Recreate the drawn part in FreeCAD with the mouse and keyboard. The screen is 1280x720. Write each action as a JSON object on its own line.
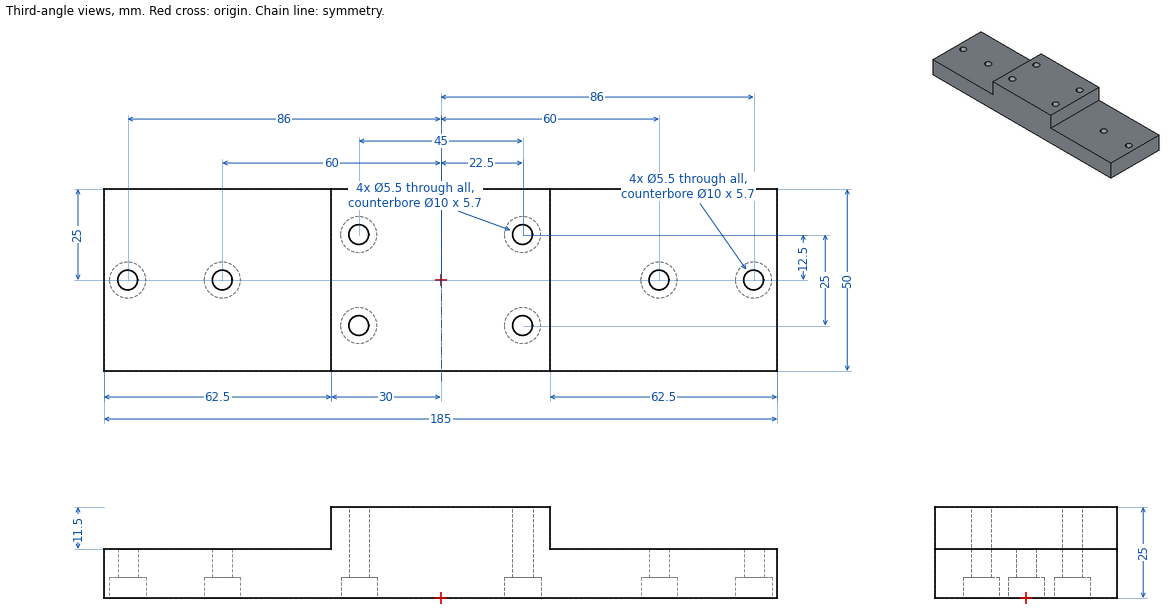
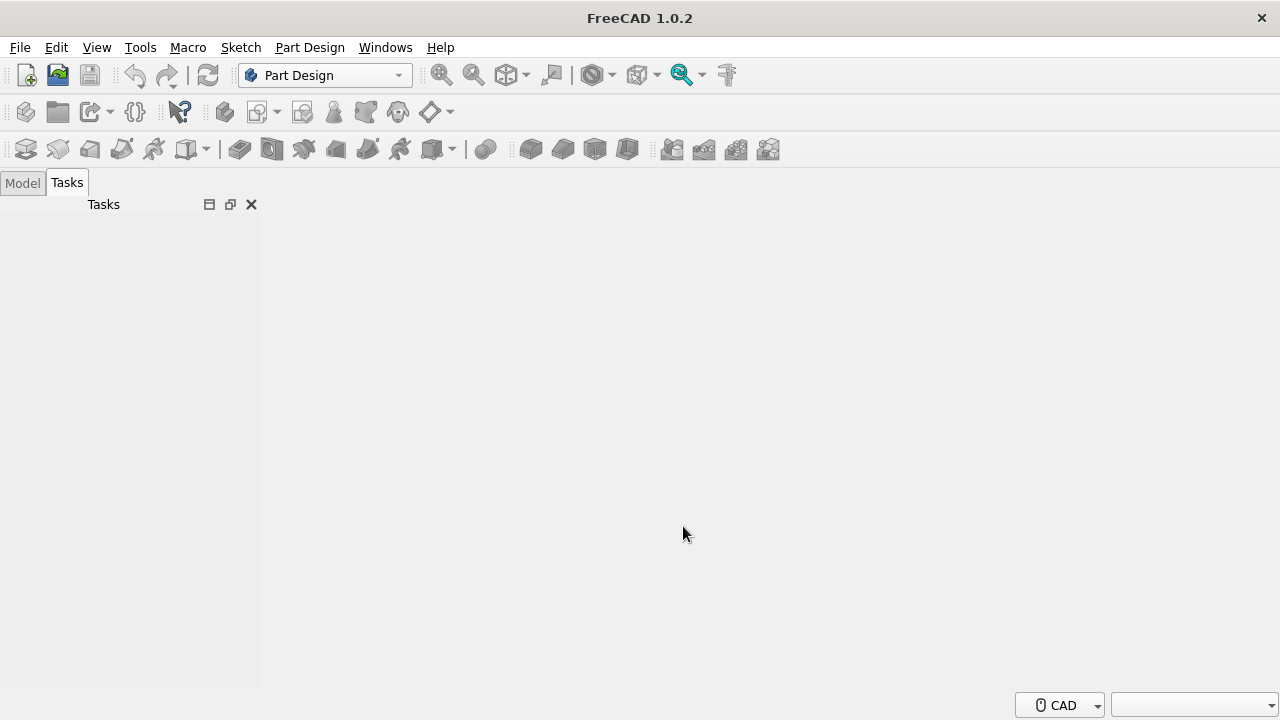
{"action": "key", "text": "ctrl+n"}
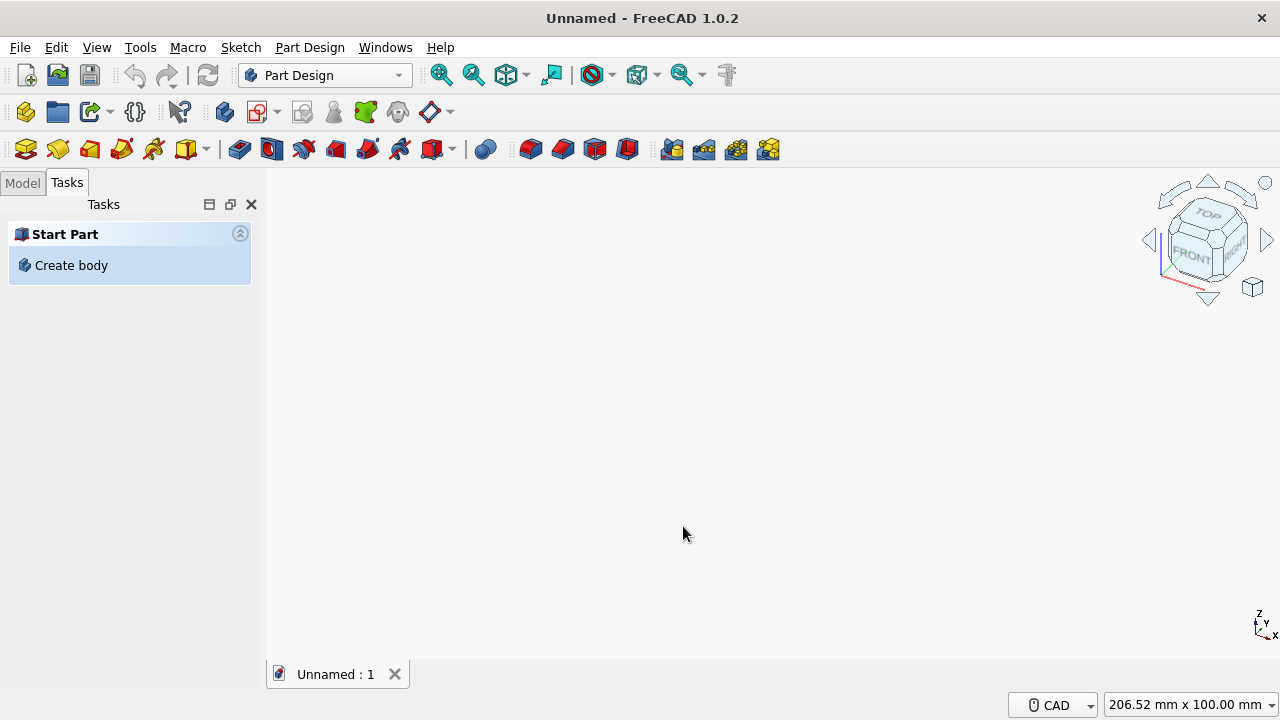
{"action": "left_click", "coordinate": [258, 112]}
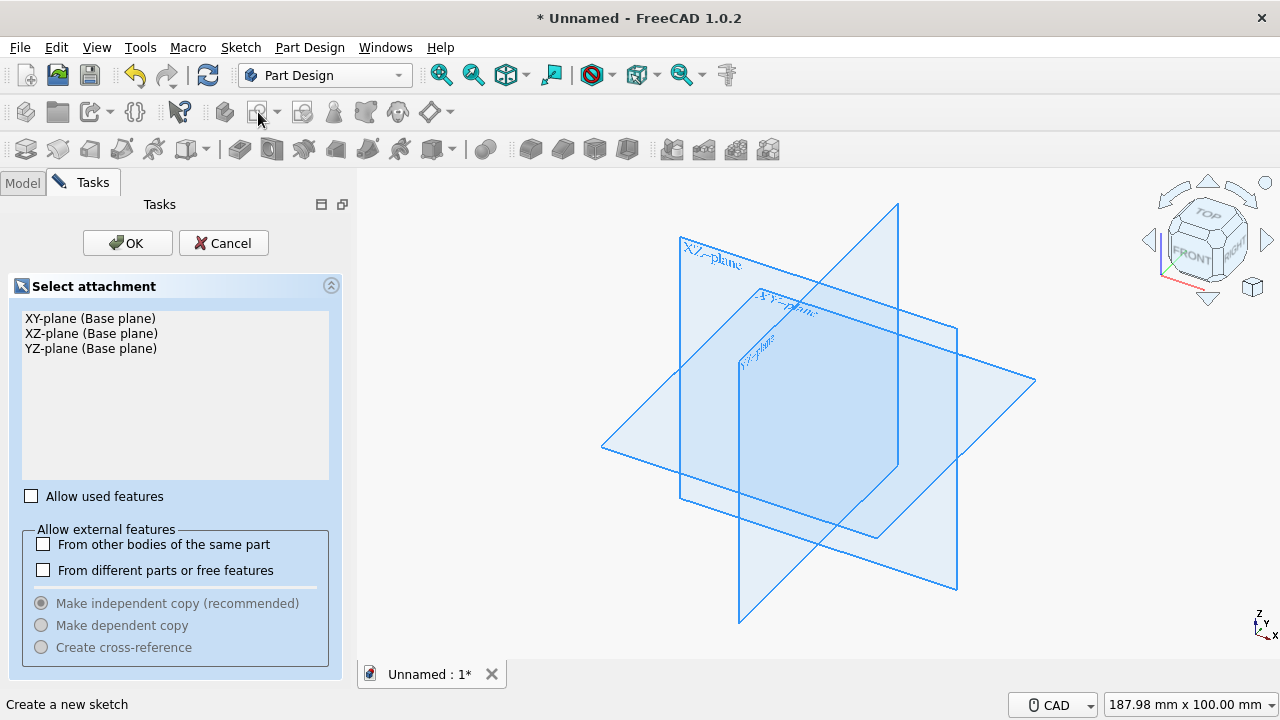
{"action": "left_click", "coordinate": [82, 318]}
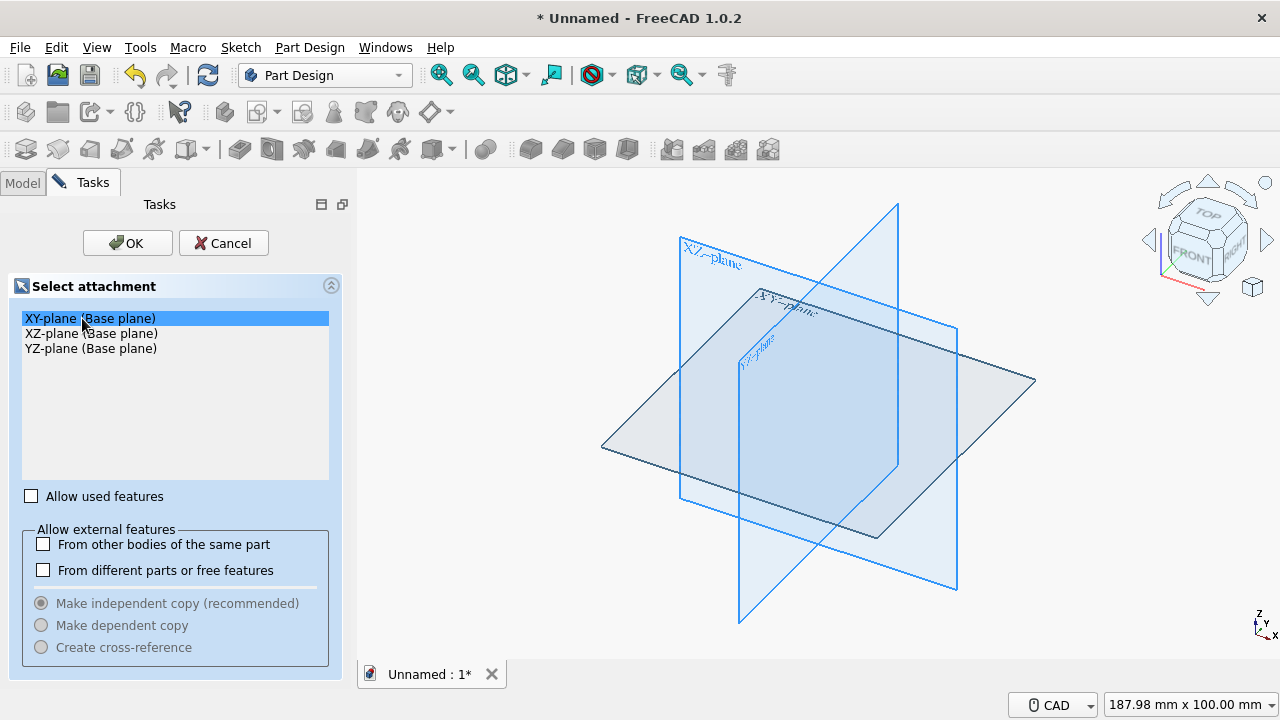
{"action": "left_click", "coordinate": [128, 243]}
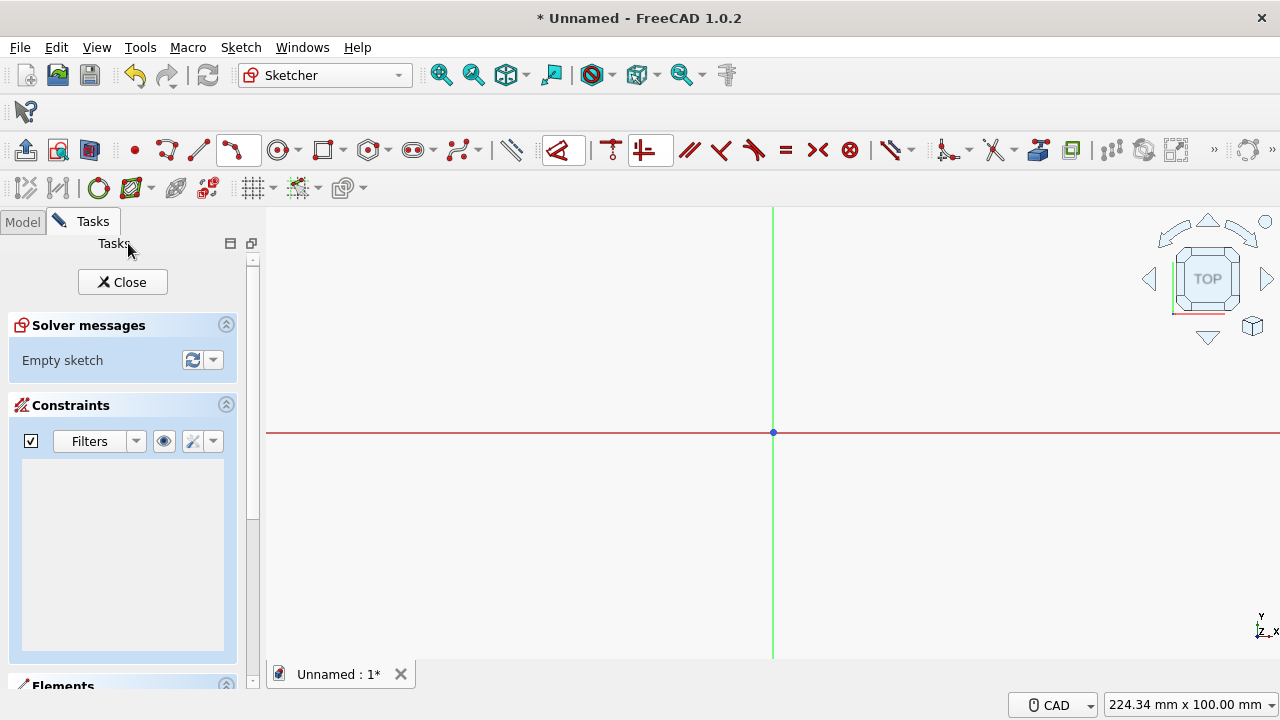
{"action": "scroll", "coordinate": [565, 433], "scroll_direction": "down", "scroll_amount": 2}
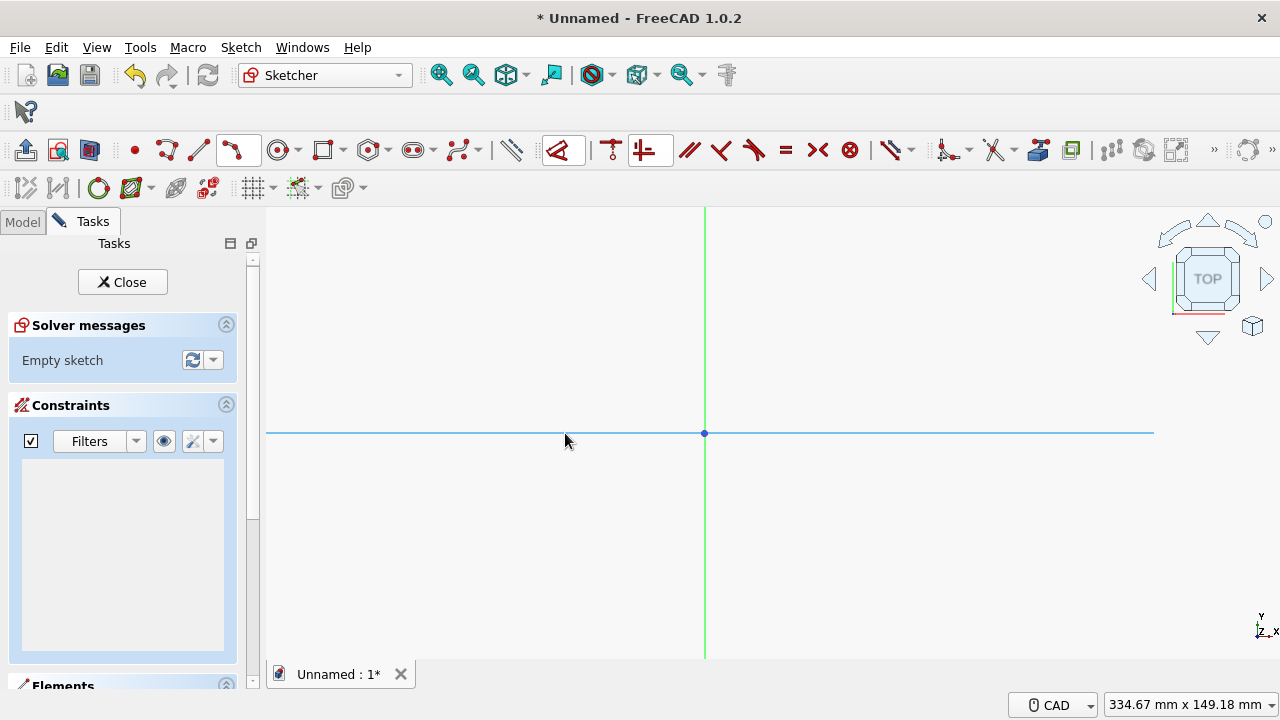
{"action": "key", "text": "g v"}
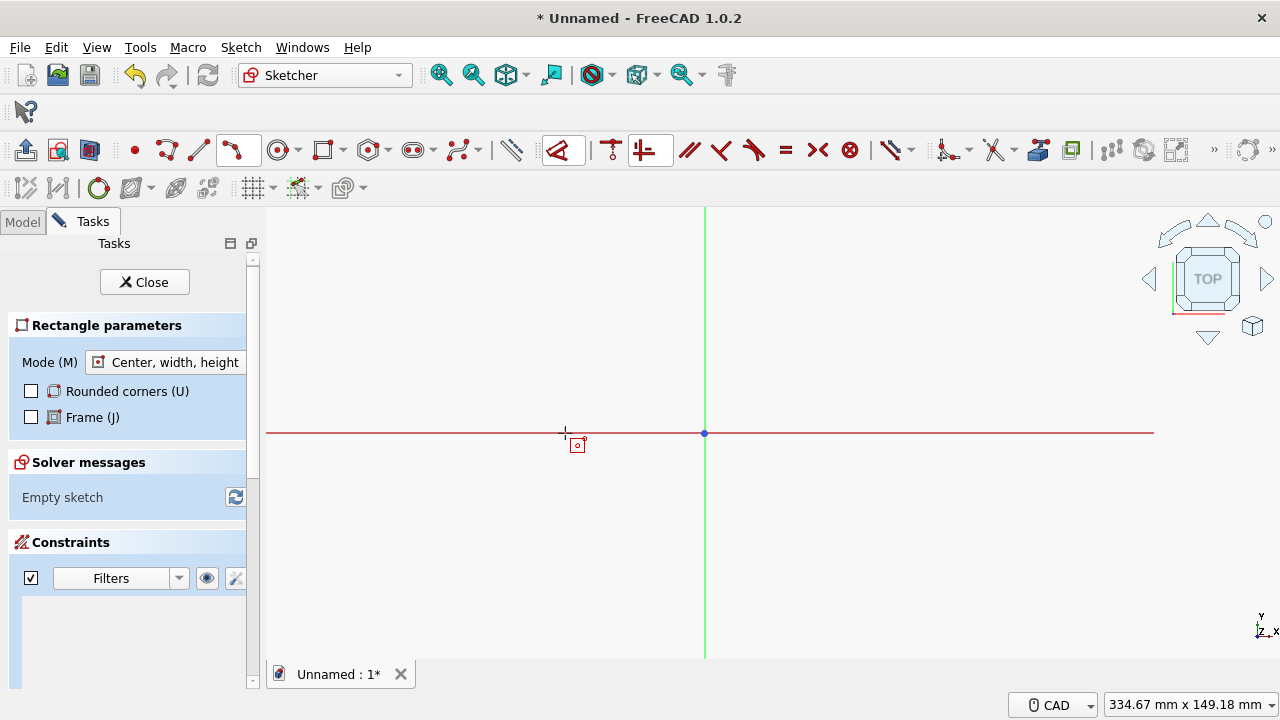
{"action": "left_click", "coordinate": [705, 433]}
{"action": "mouse_move", "coordinate": [985, 357]}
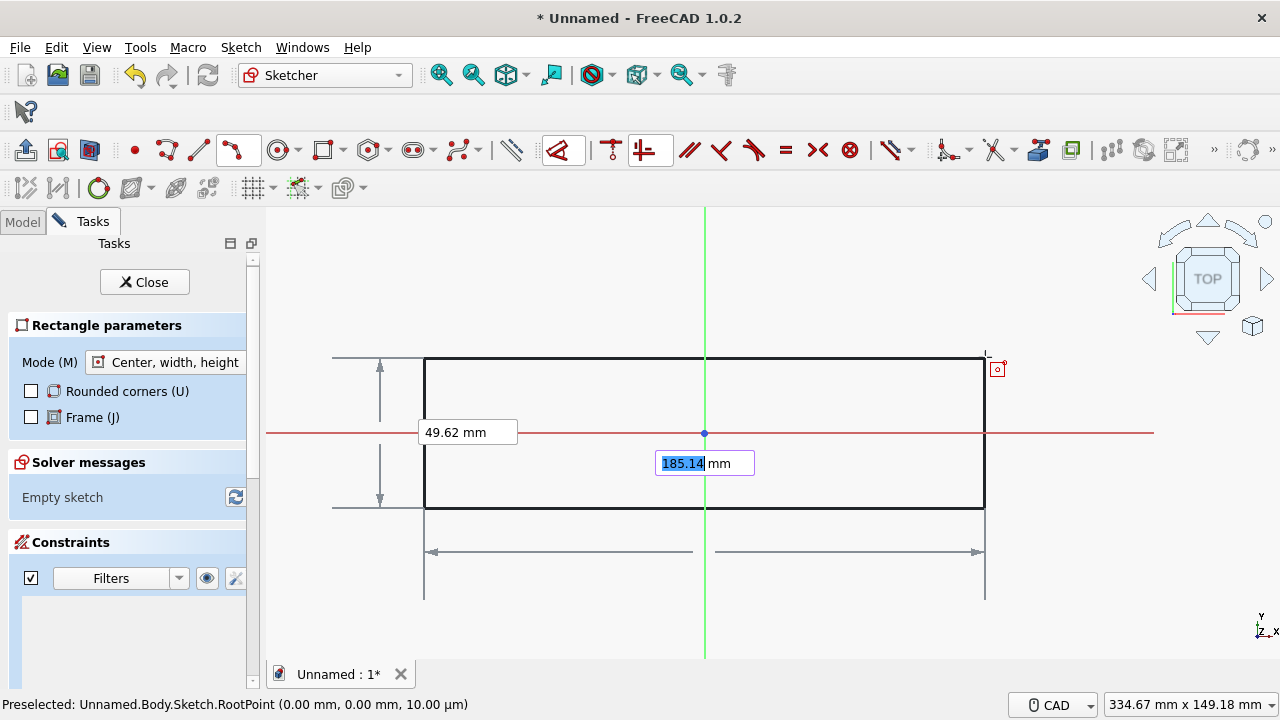
{"action": "type", "text": "185"}
{"action": "key", "text": "Tab"}
{"action": "type", "text": "50"}
{"action": "key", "text": "Return"}
{"action": "key", "text": "Escape"}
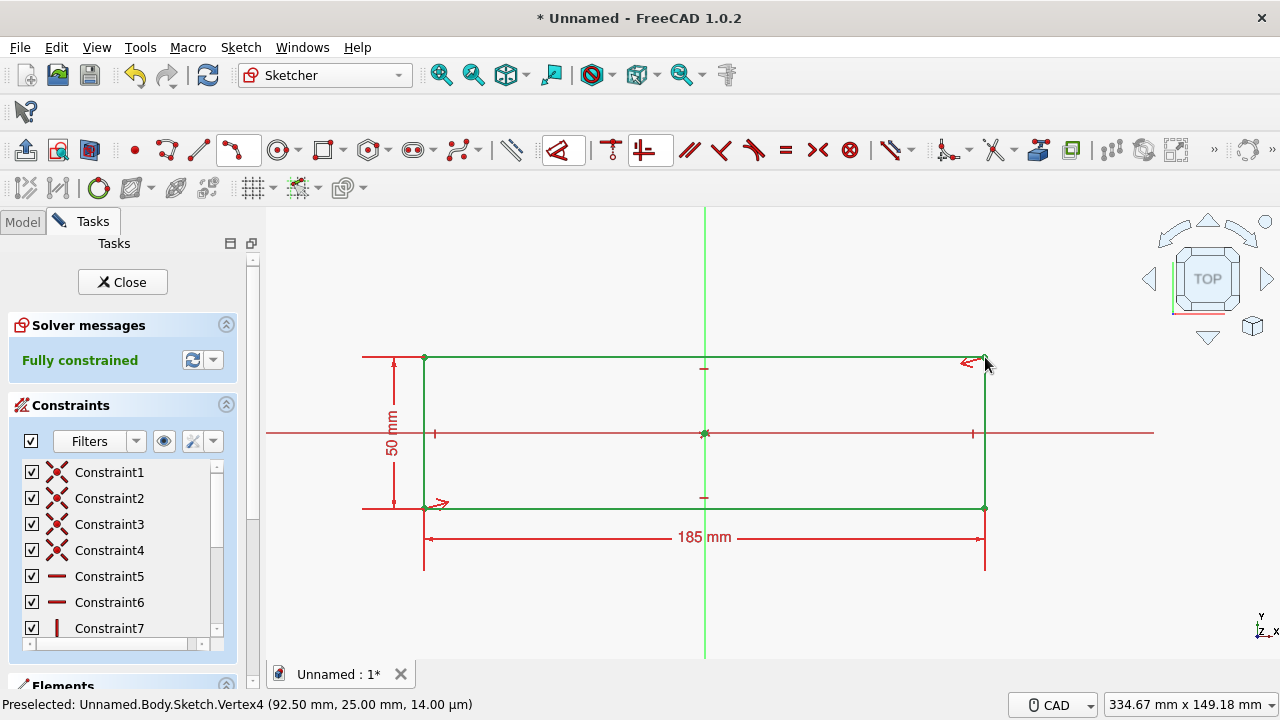
{"action": "left_click", "coordinate": [123, 282]}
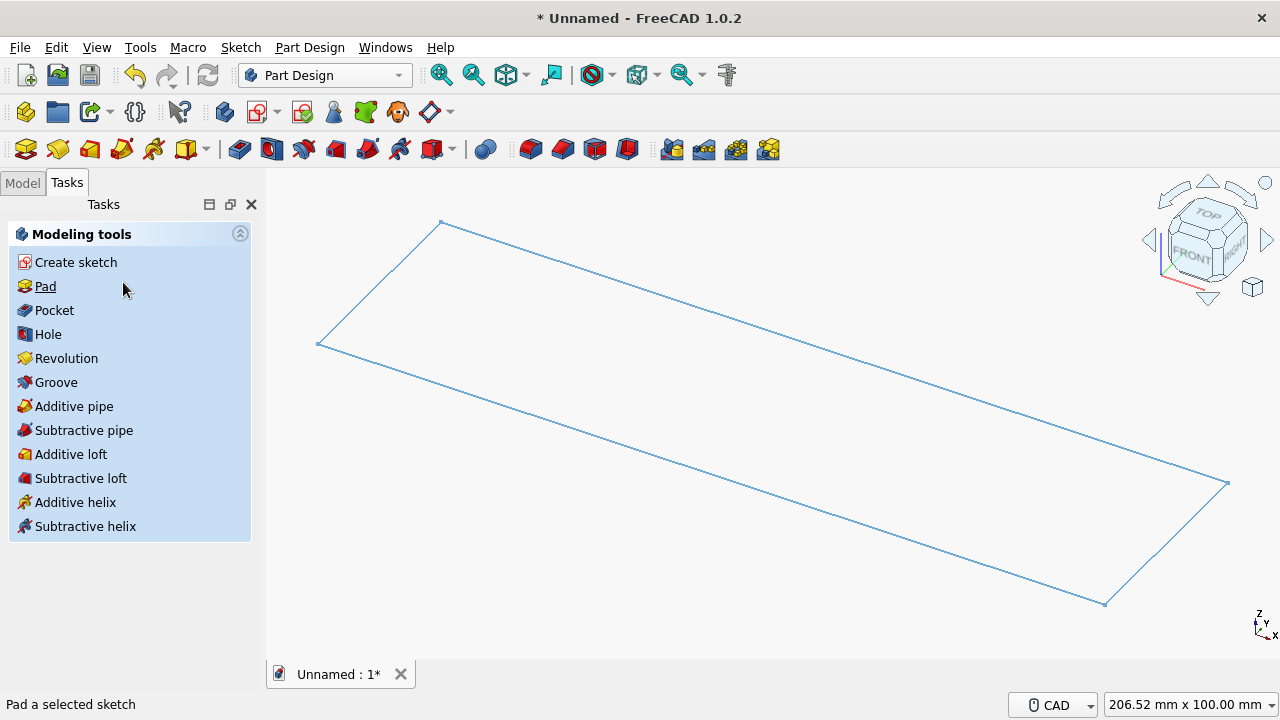
{"action": "left_click", "coordinate": [26, 150]}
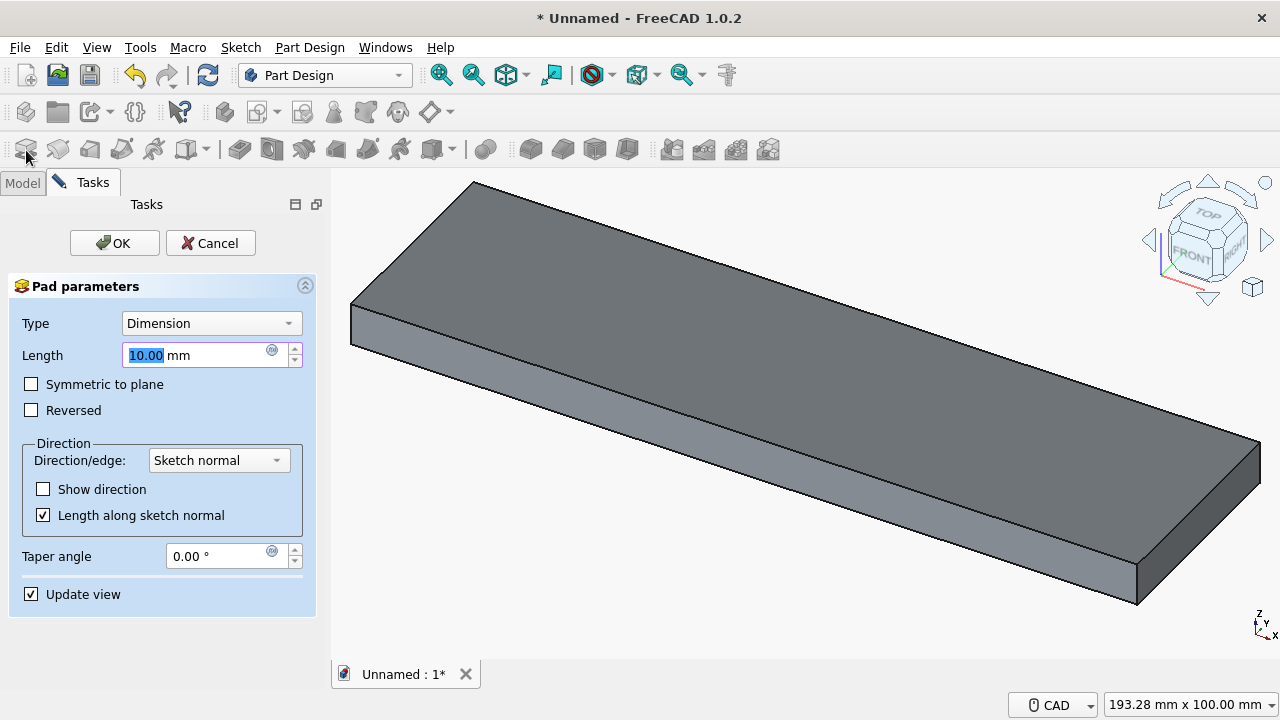
{"action": "type", "text": "25"}
{"action": "key", "text": "Tab"}